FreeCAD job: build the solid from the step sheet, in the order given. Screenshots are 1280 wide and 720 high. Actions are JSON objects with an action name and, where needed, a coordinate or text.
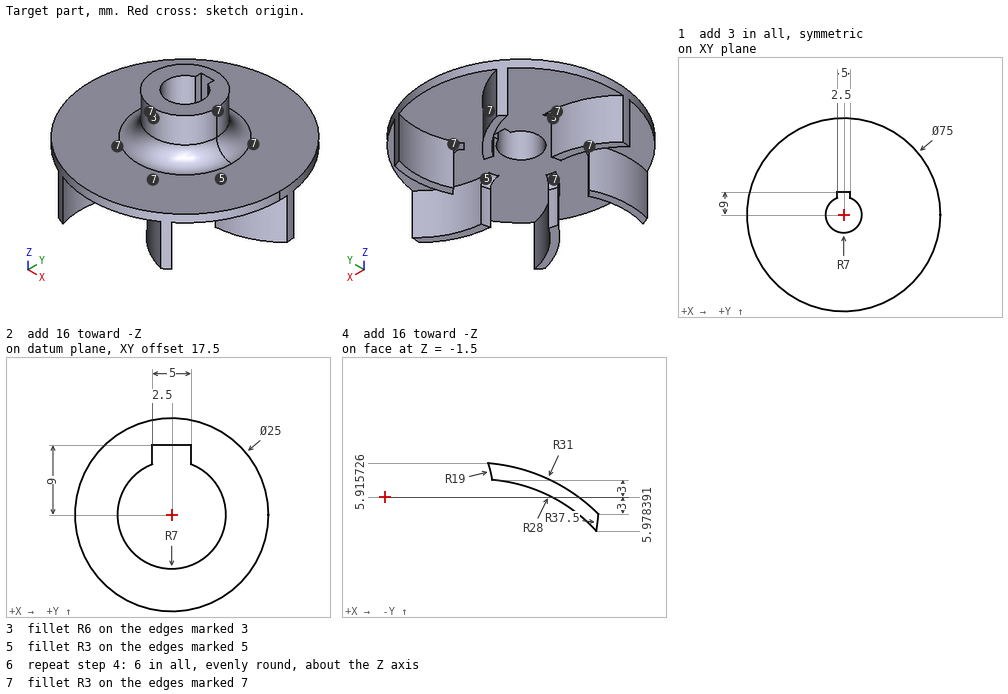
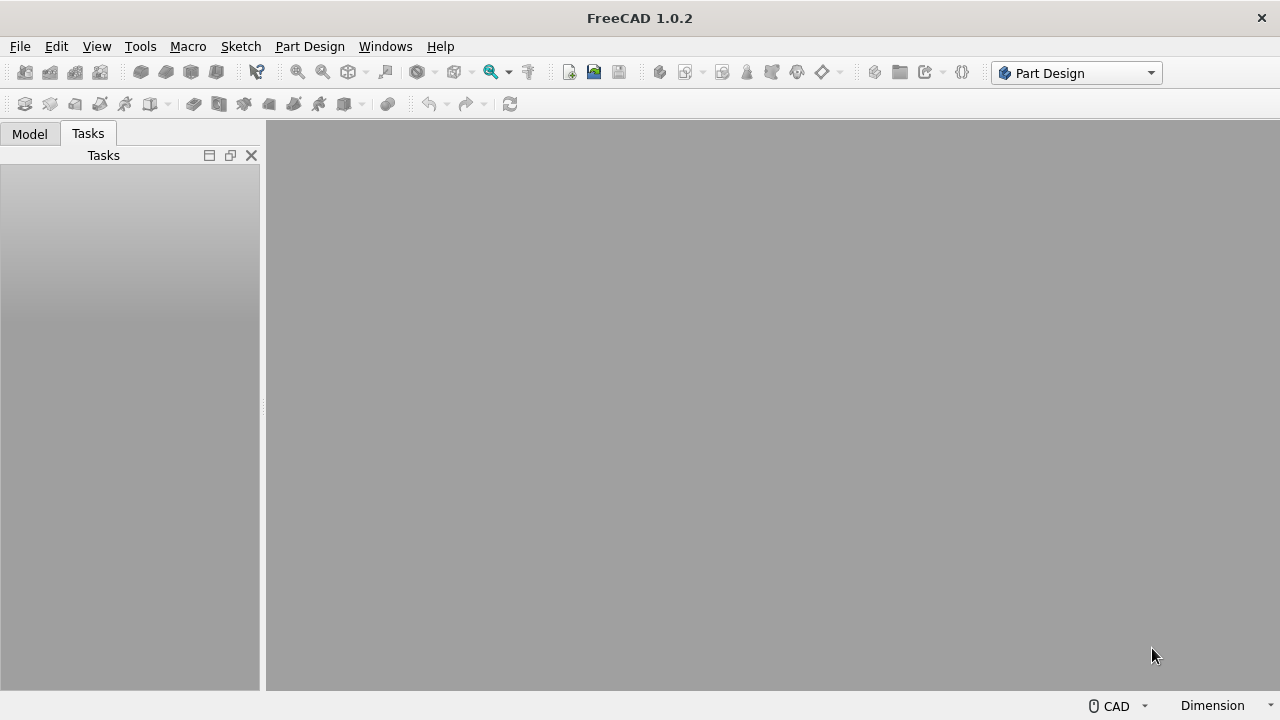
{"action": "left_click", "coordinate": [569, 72]}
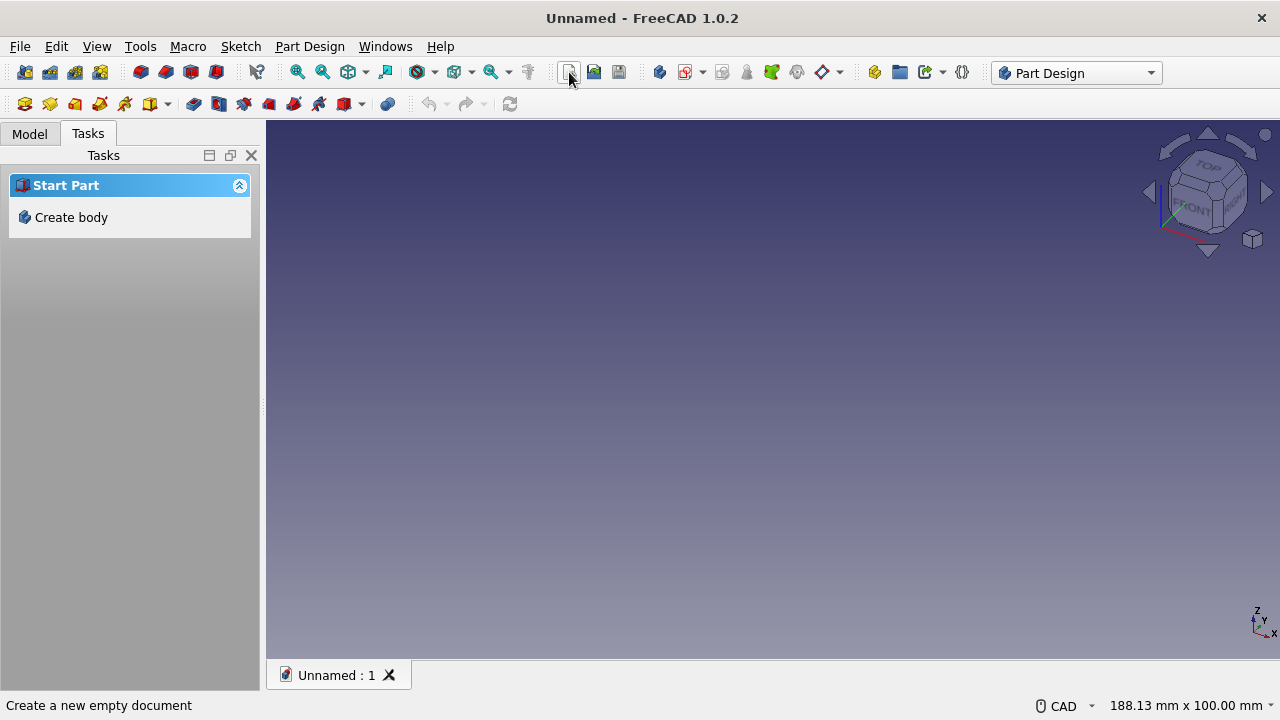
{"action": "left_click", "coordinate": [684, 72]}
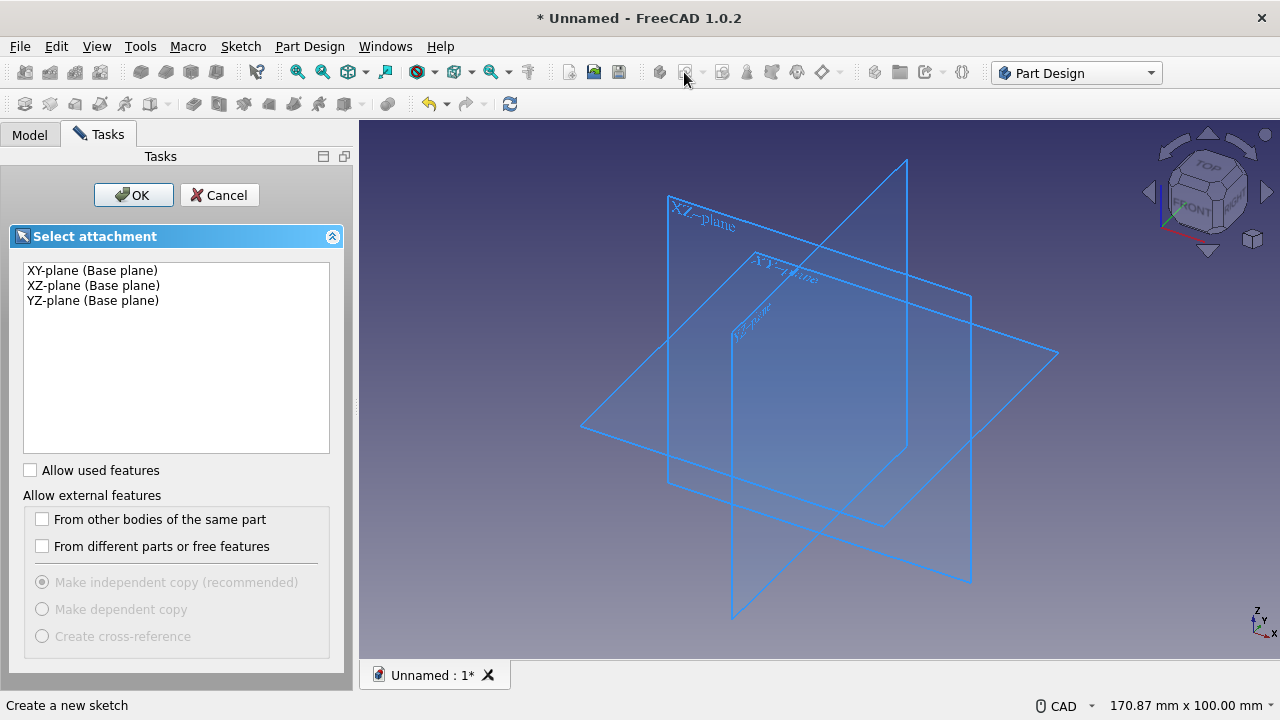
{"action": "left_click", "coordinate": [84, 270]}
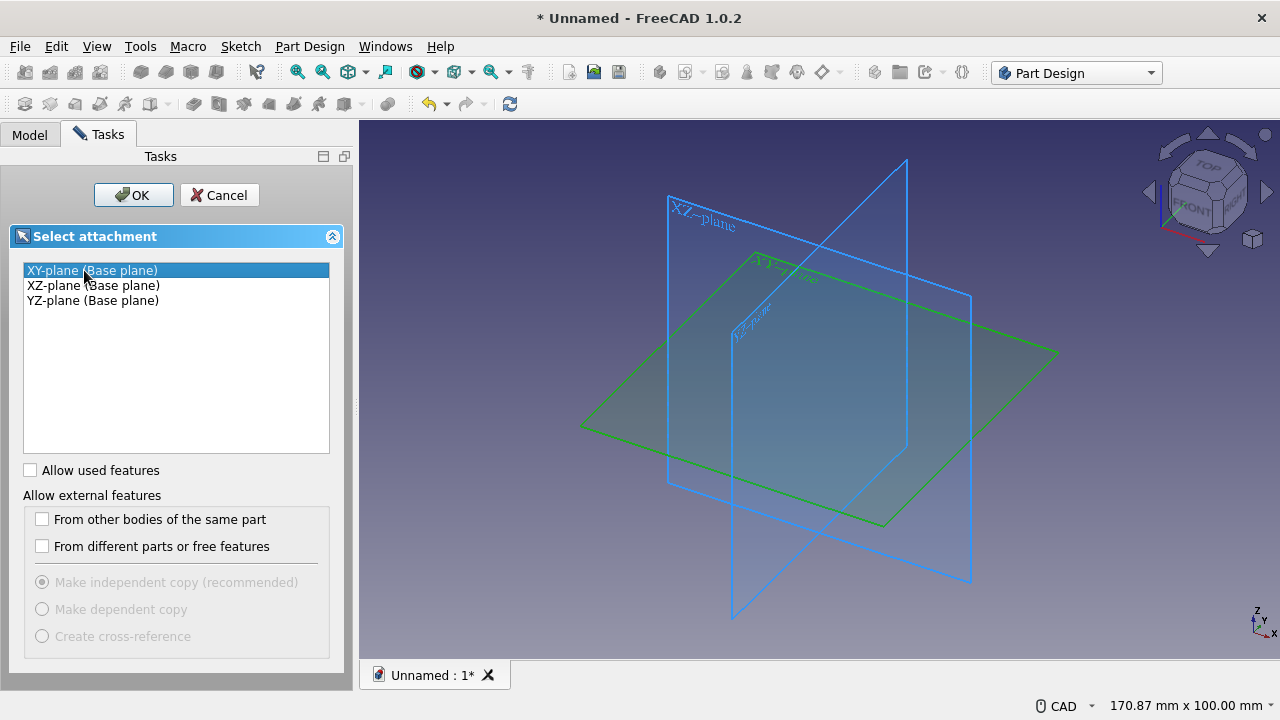
{"action": "left_click", "coordinate": [134, 195]}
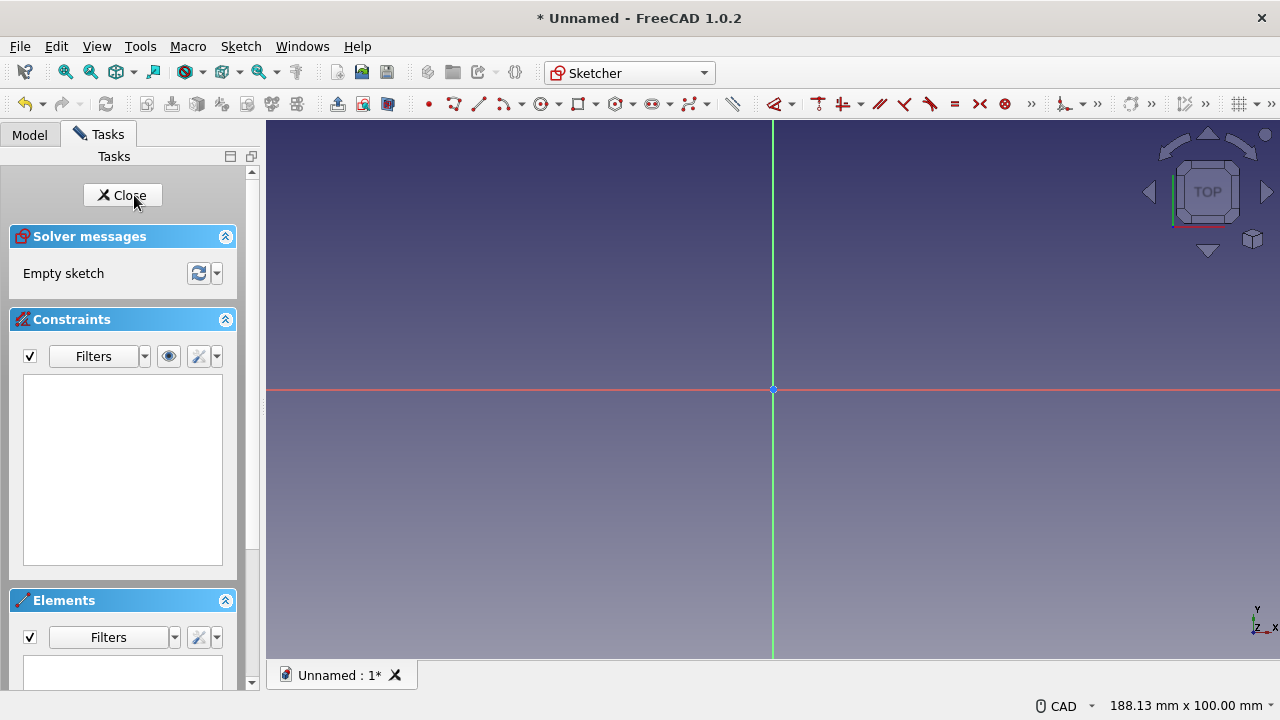
{"action": "left_click", "coordinate": [454, 104]}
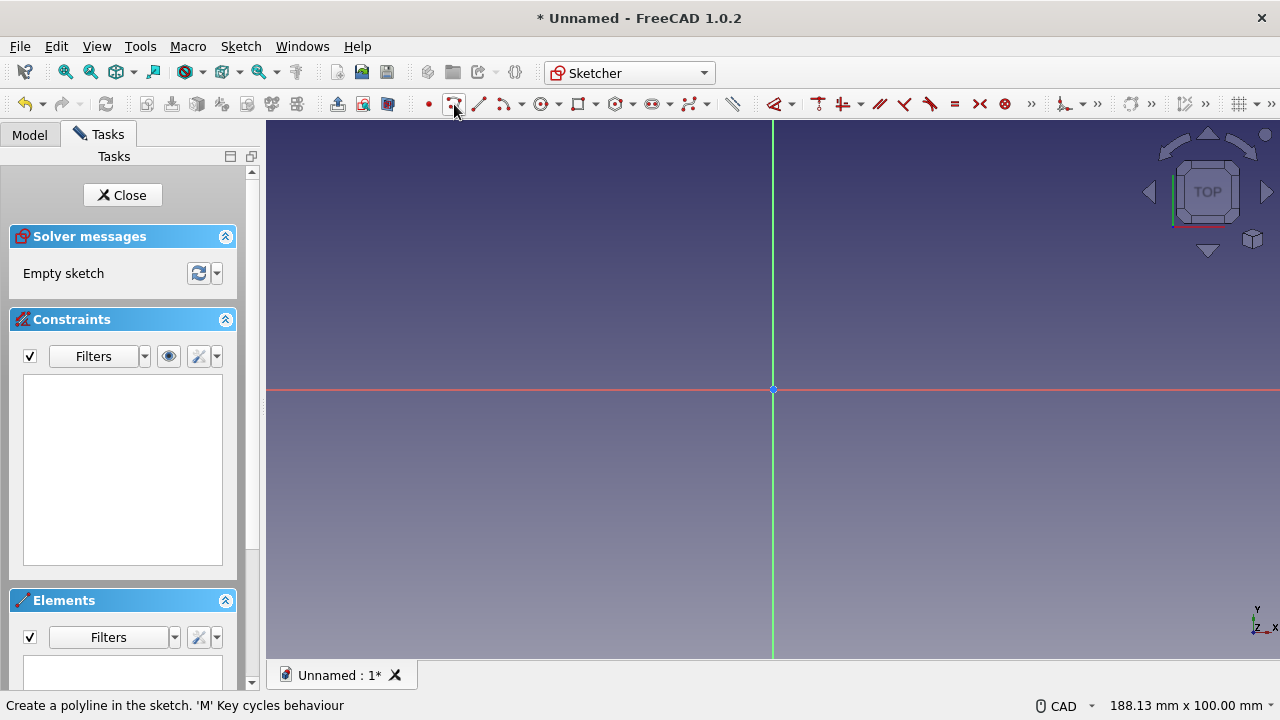
{"action": "left_click", "coordinate": [760, 354]}
{"action": "left_click", "coordinate": [760, 341]}
{"action": "left_click", "coordinate": [786, 341]}
{"action": "left_click", "coordinate": [786, 354]}
{"action": "right_click", "coordinate": [786, 354]}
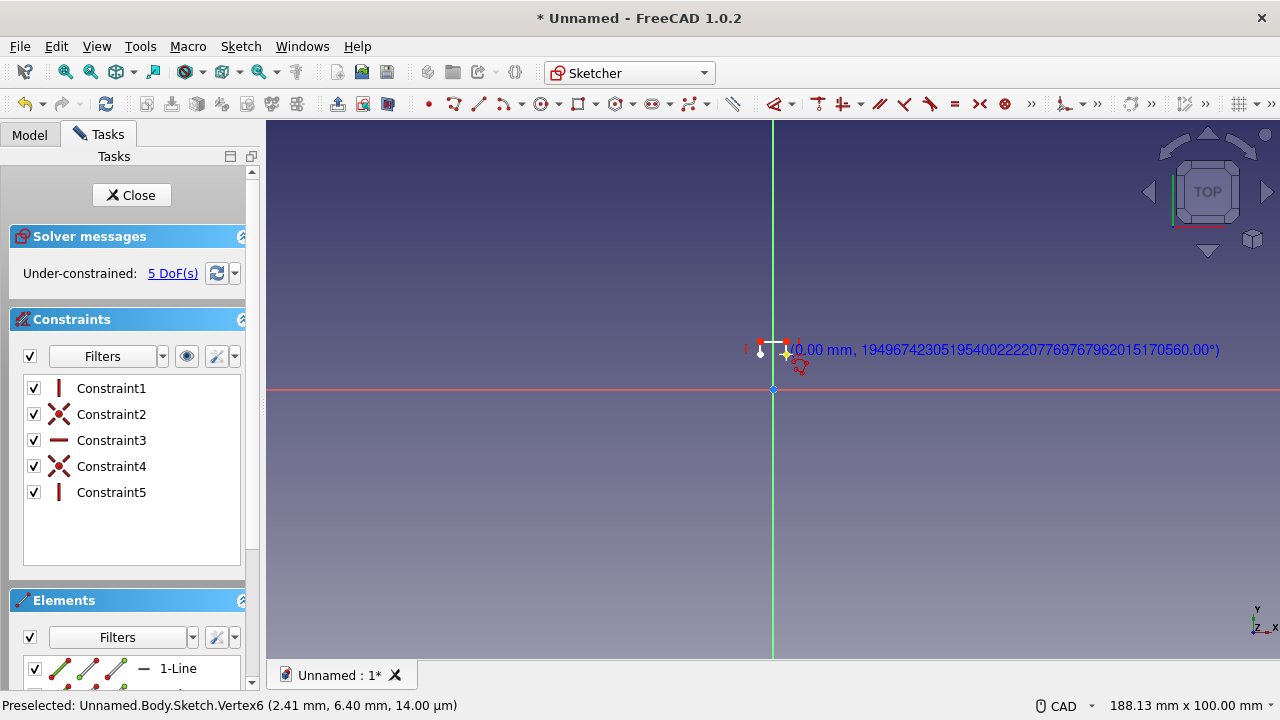
{"action": "left_click", "coordinate": [522, 104]}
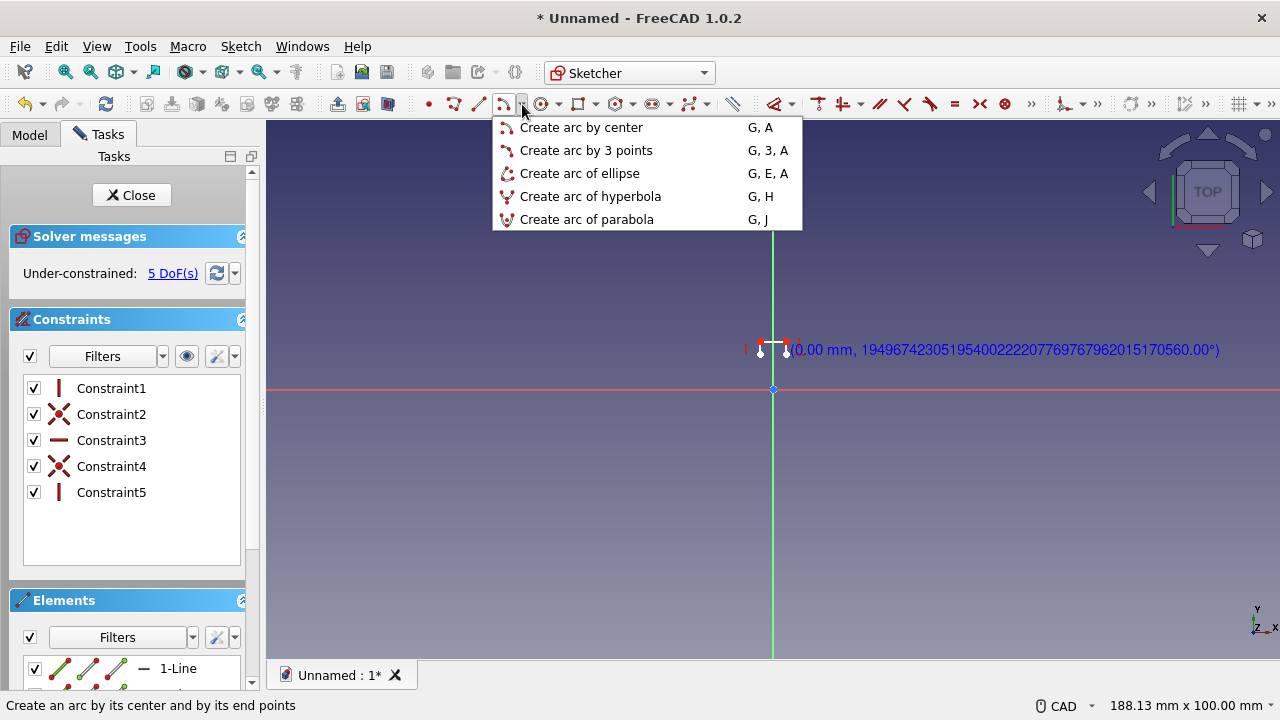
{"action": "left_click", "coordinate": [648, 150]}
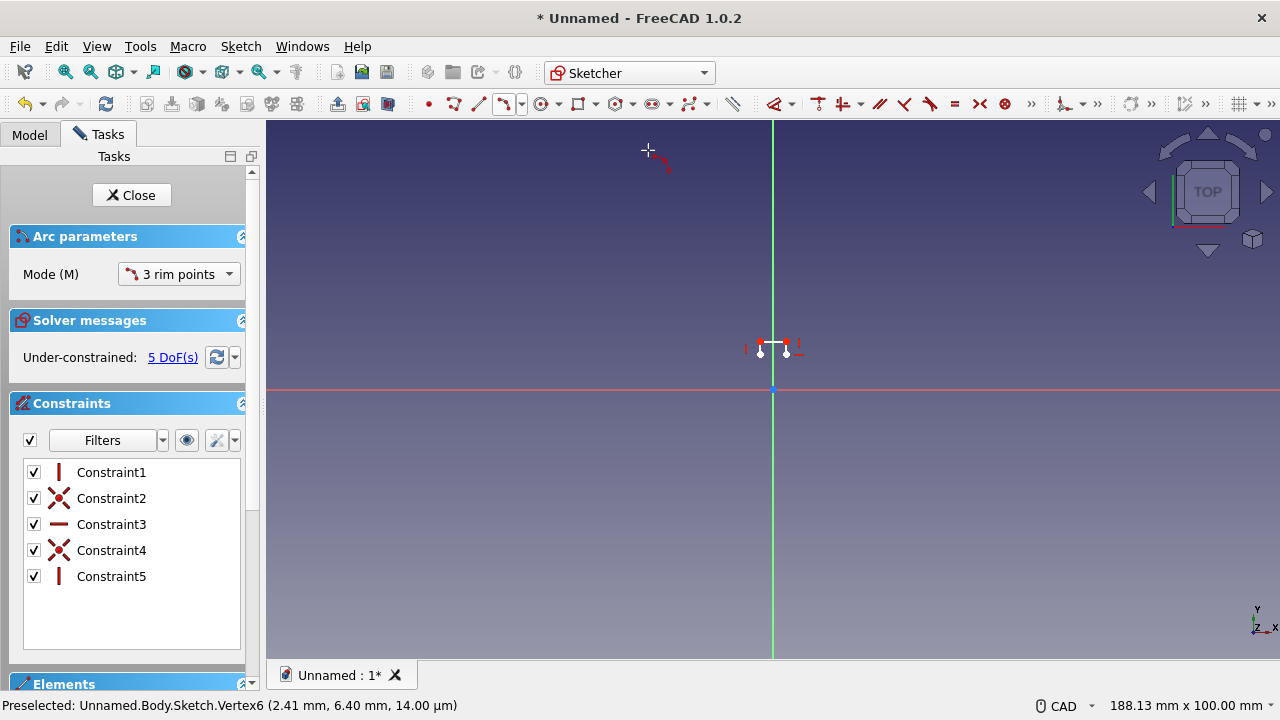
{"action": "scroll", "coordinate": [786, 354], "scroll_direction": "up", "scroll_amount": 5}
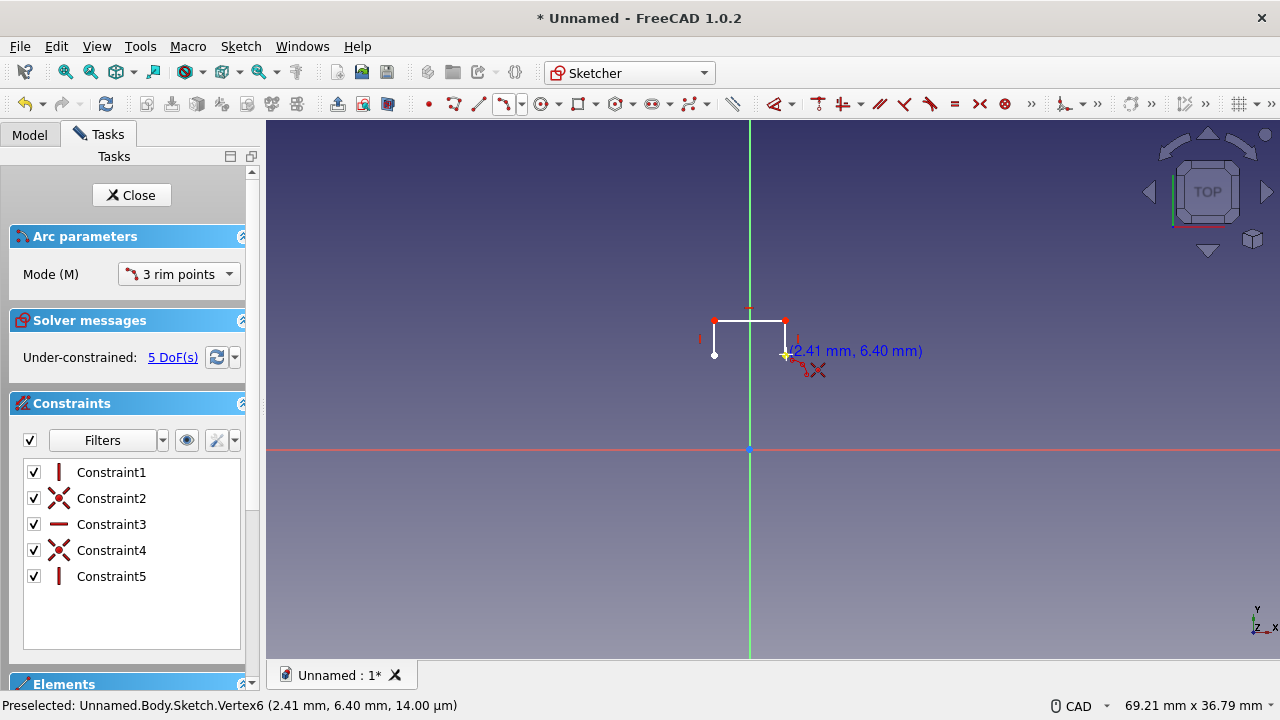
{"action": "left_click", "coordinate": [785, 356]}
{"action": "left_click", "coordinate": [714, 356]}
{"action": "left_click", "coordinate": [696, 537]}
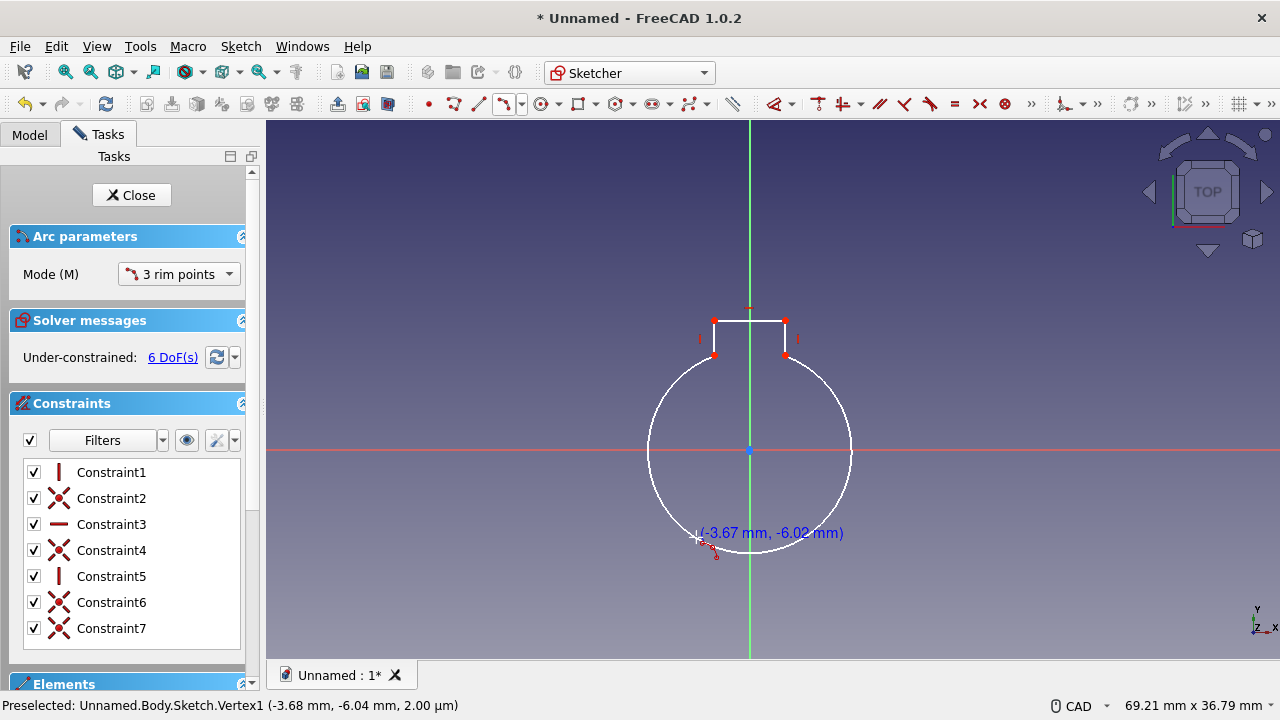
{"action": "left_click", "coordinate": [540, 104]}